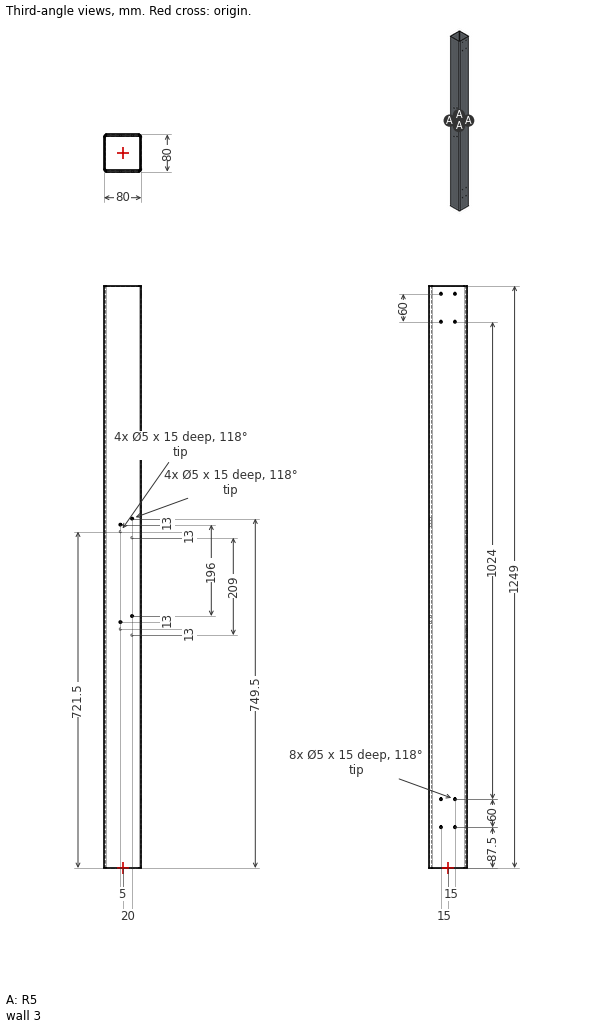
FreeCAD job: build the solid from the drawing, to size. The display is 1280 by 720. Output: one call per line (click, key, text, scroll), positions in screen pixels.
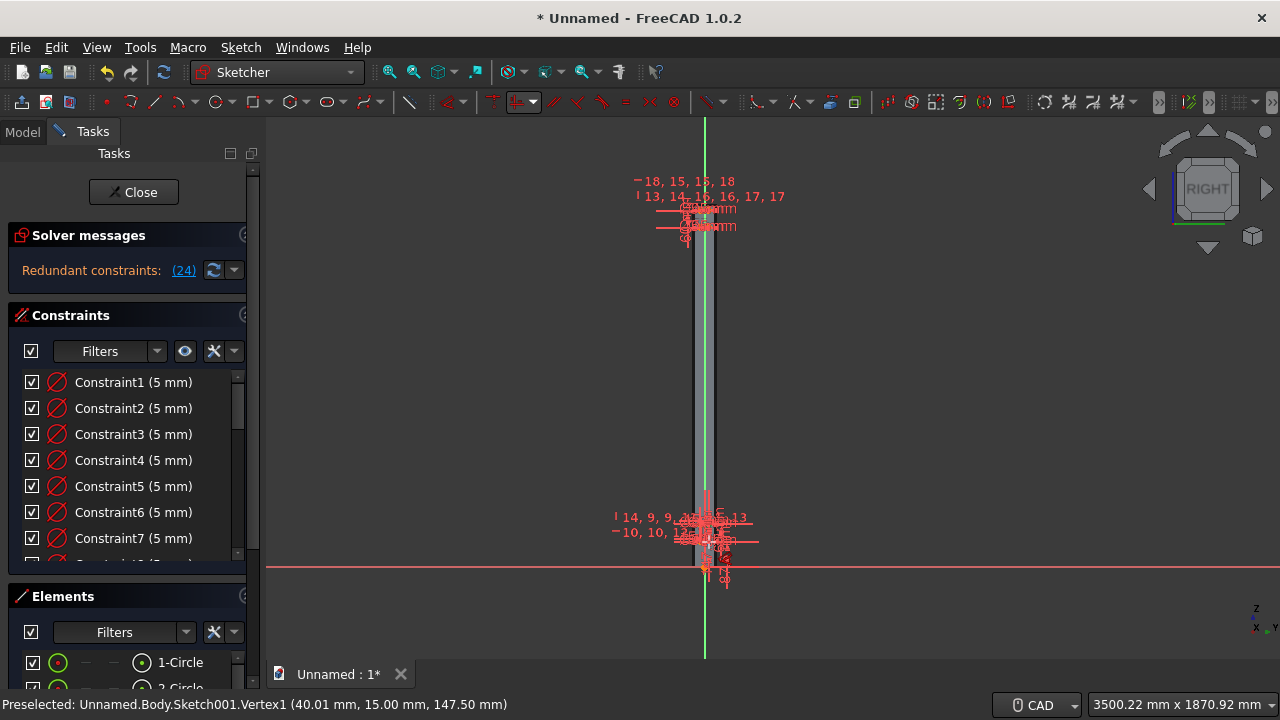
scroll(709, 228, up, 2)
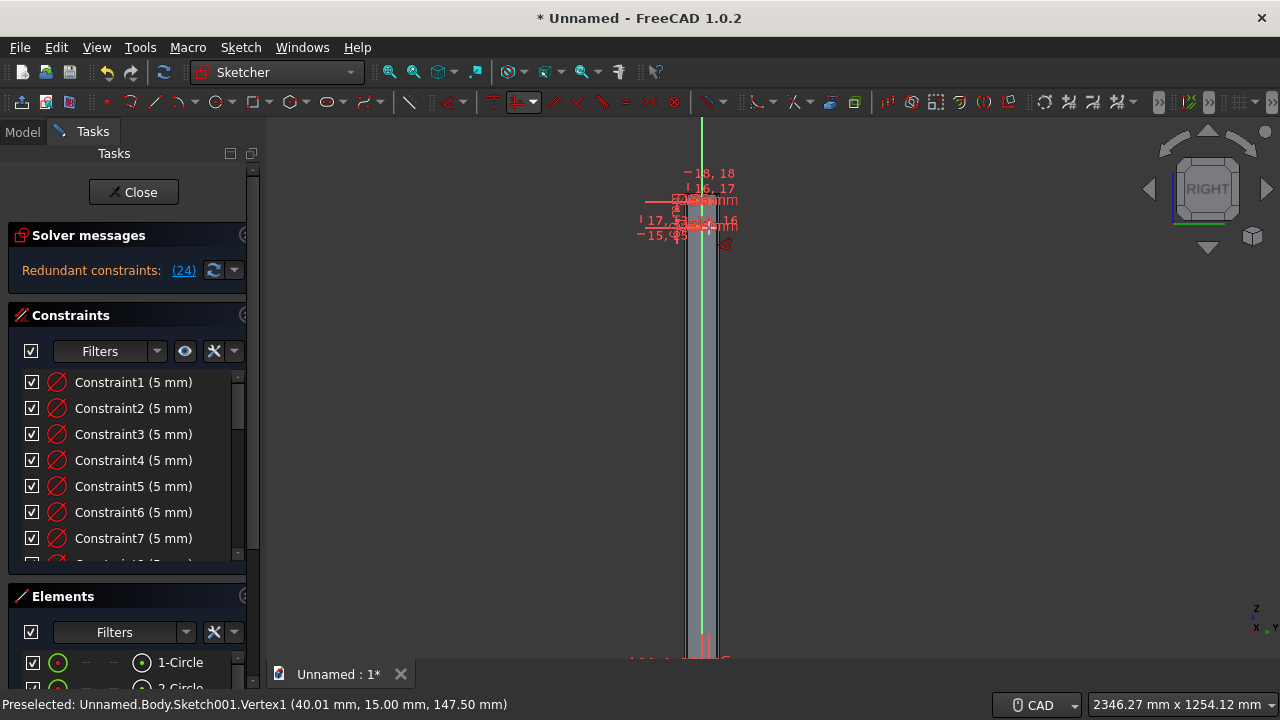
click(709, 228)
click(743, 429)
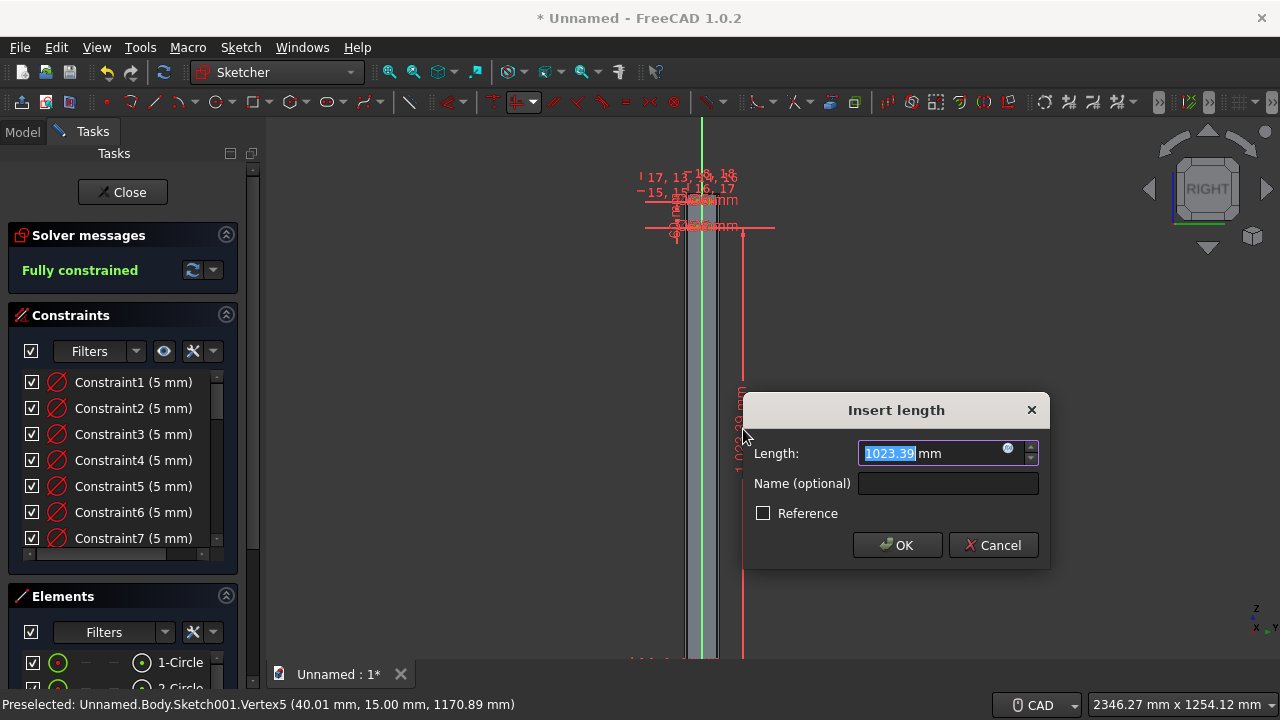
text(1024)
key(Return)
key(Escape)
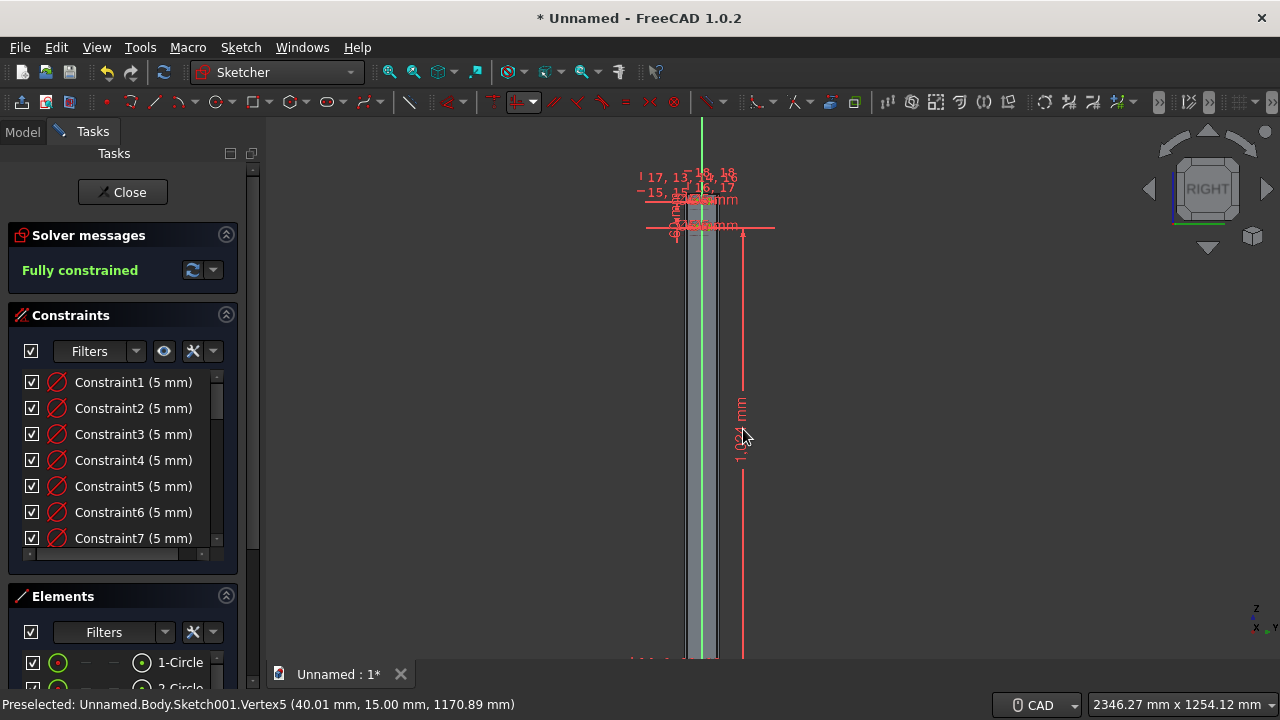
click(123, 192)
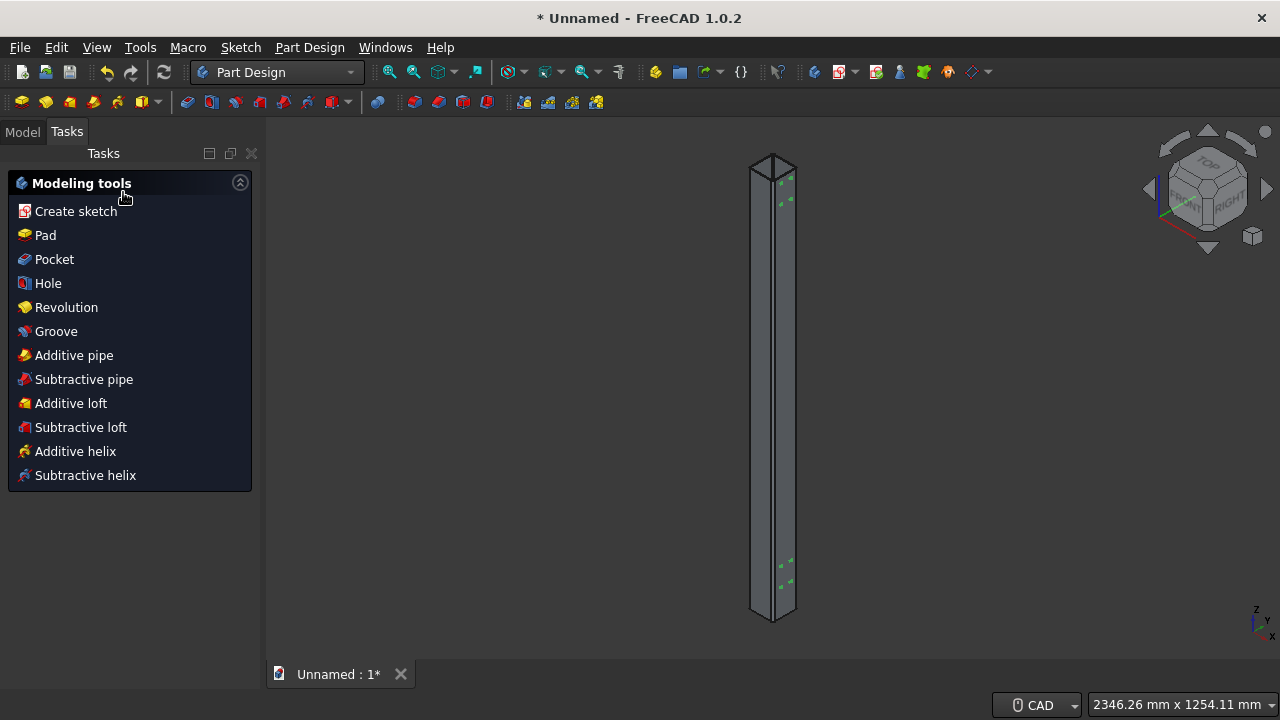
click(212, 102)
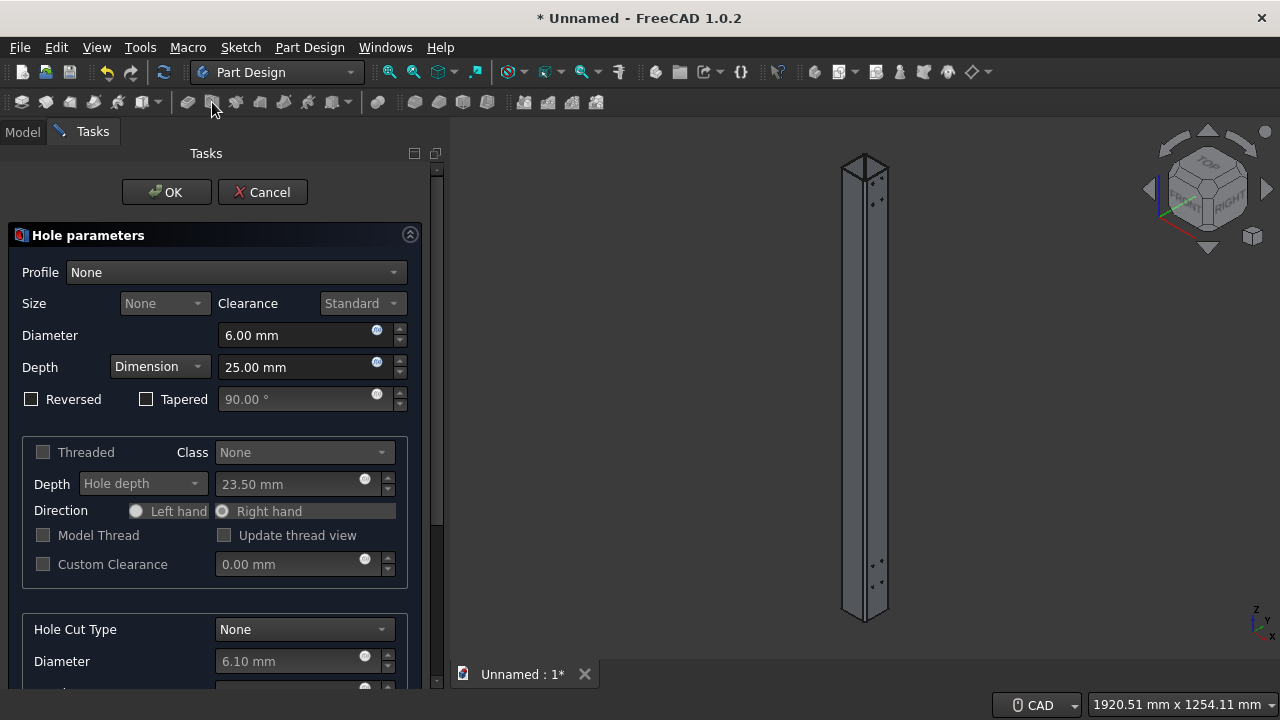
triple_click(305, 335)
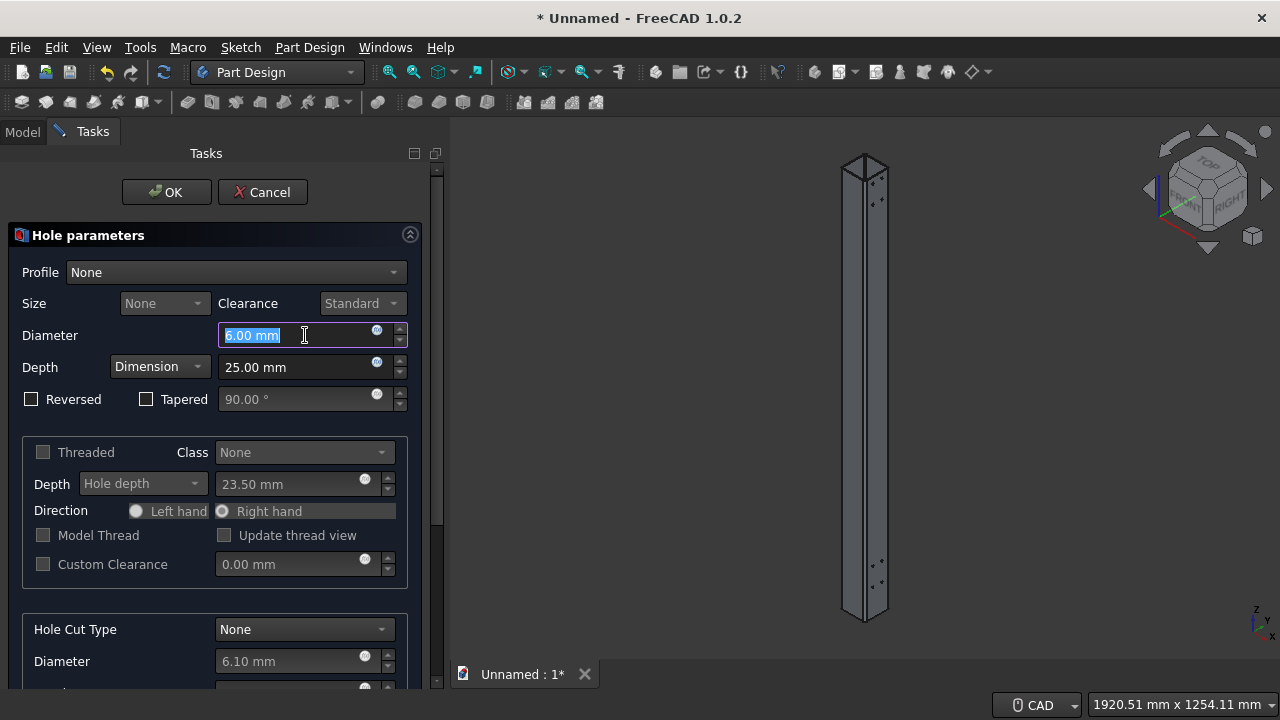
text(5)
key(Tab)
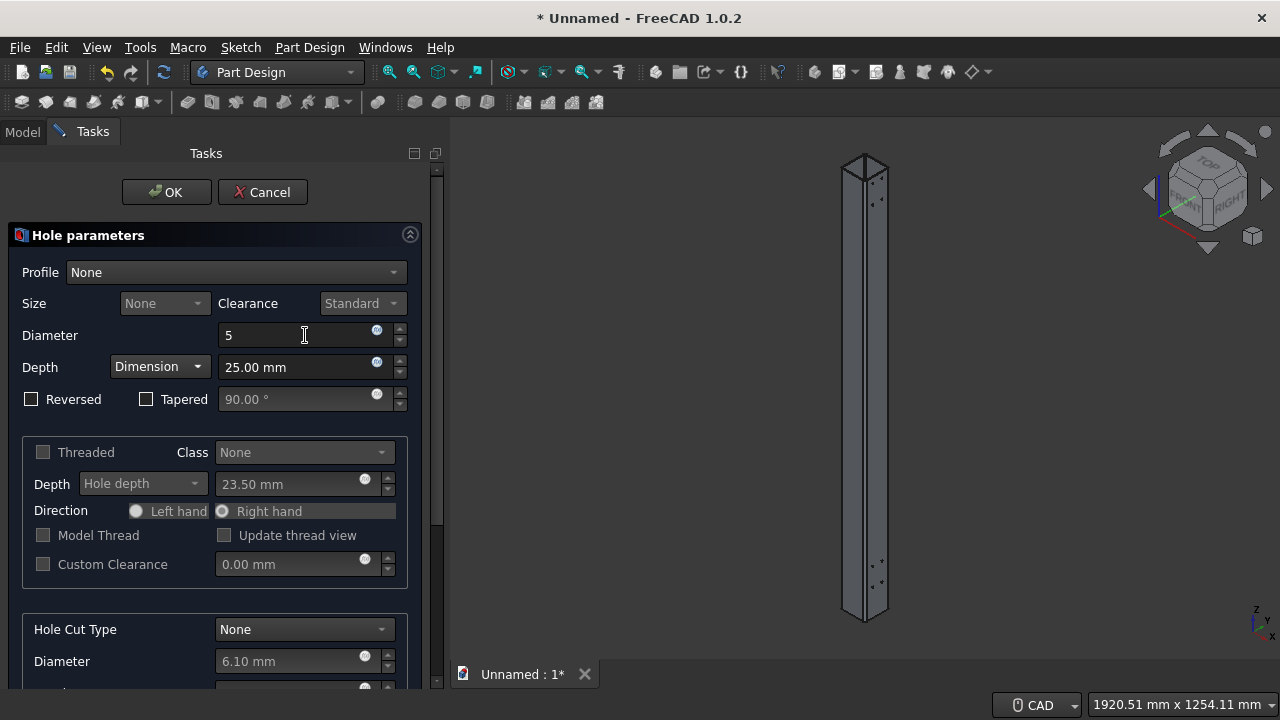
triple_click(305, 367)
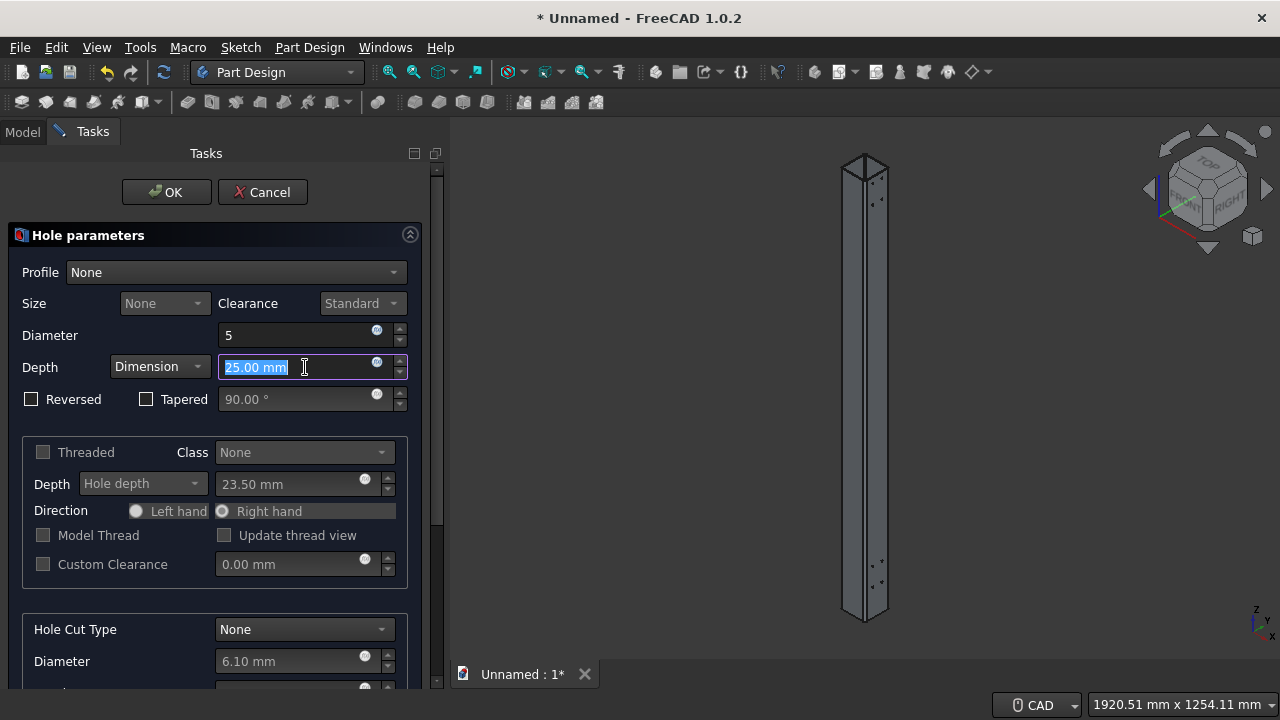
text(15)
key(Tab)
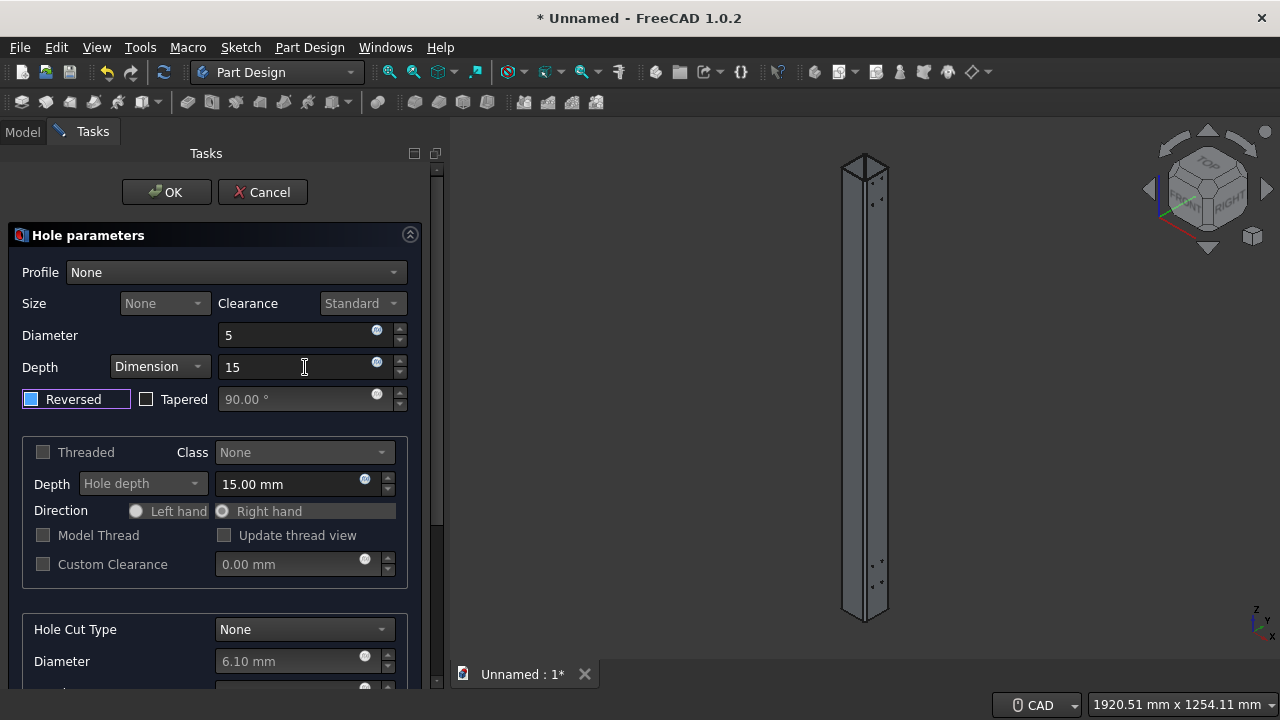
click(167, 192)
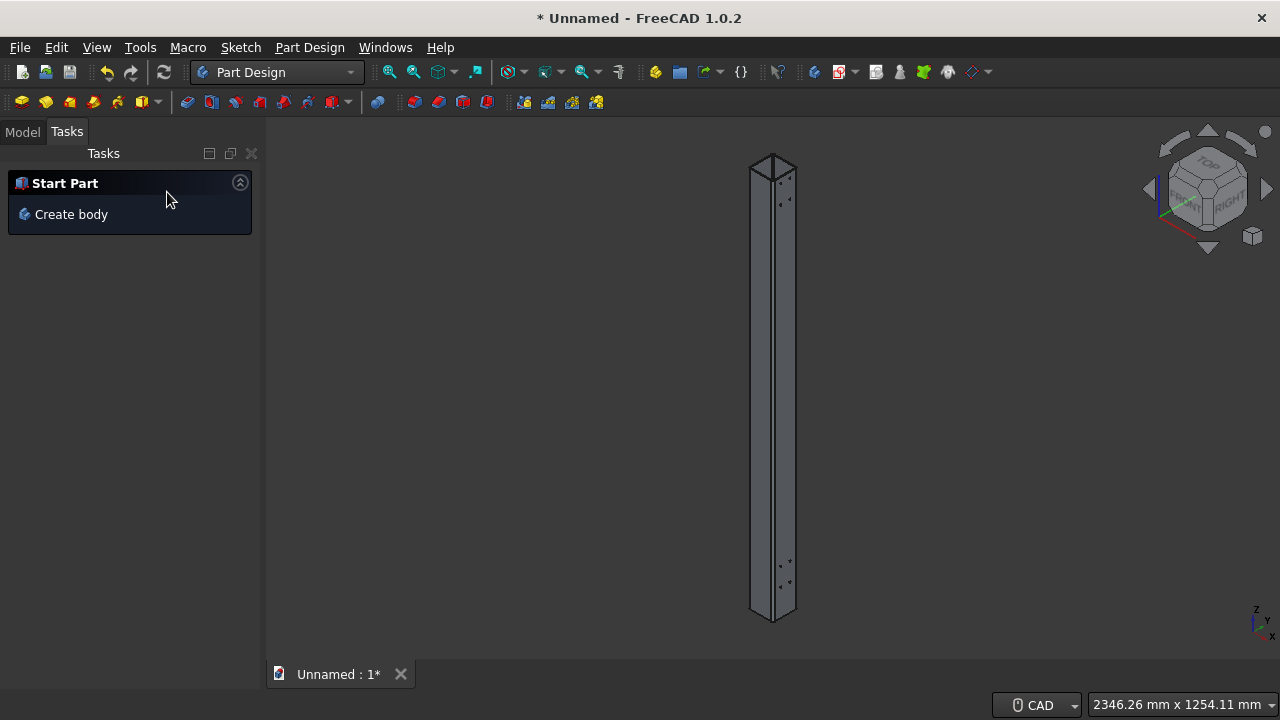
click(761, 205)